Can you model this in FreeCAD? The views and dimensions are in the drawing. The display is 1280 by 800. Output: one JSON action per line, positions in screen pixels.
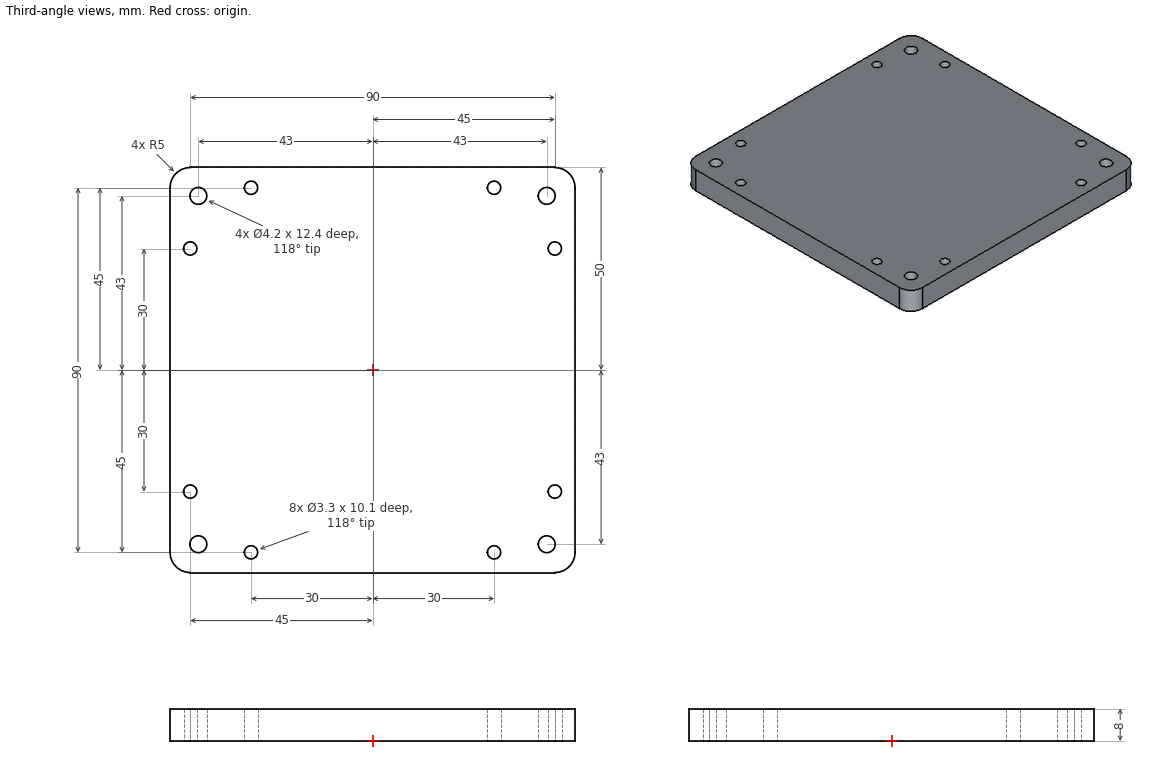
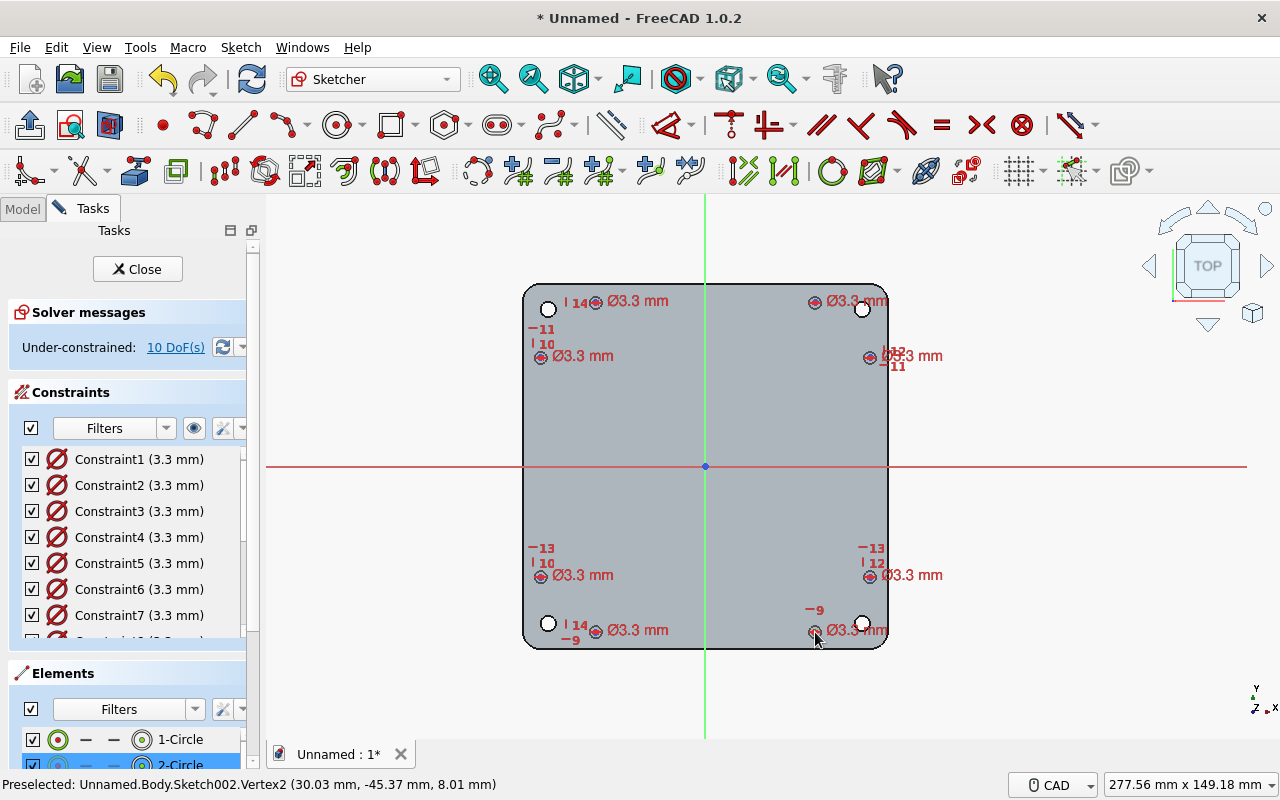
{"action": "left_click", "coordinate": [815, 303]}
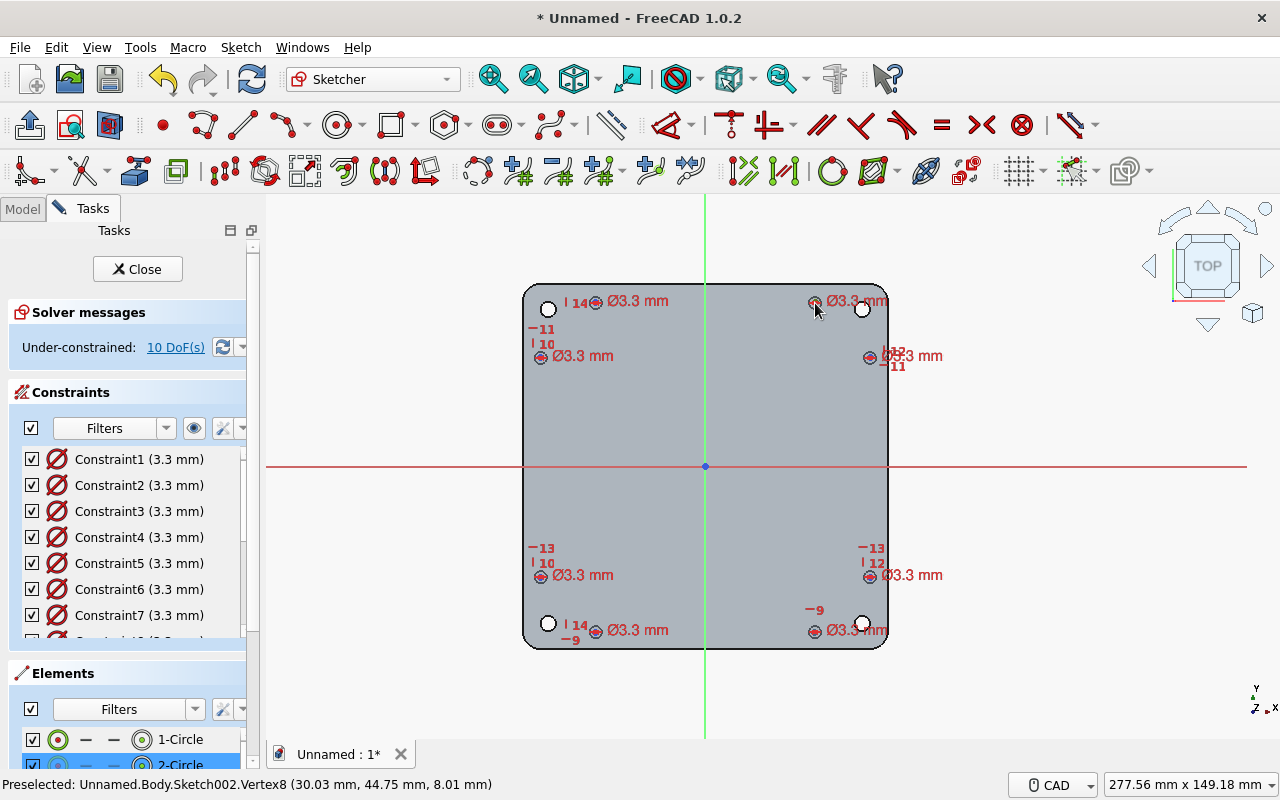
{"action": "key", "text": "v"}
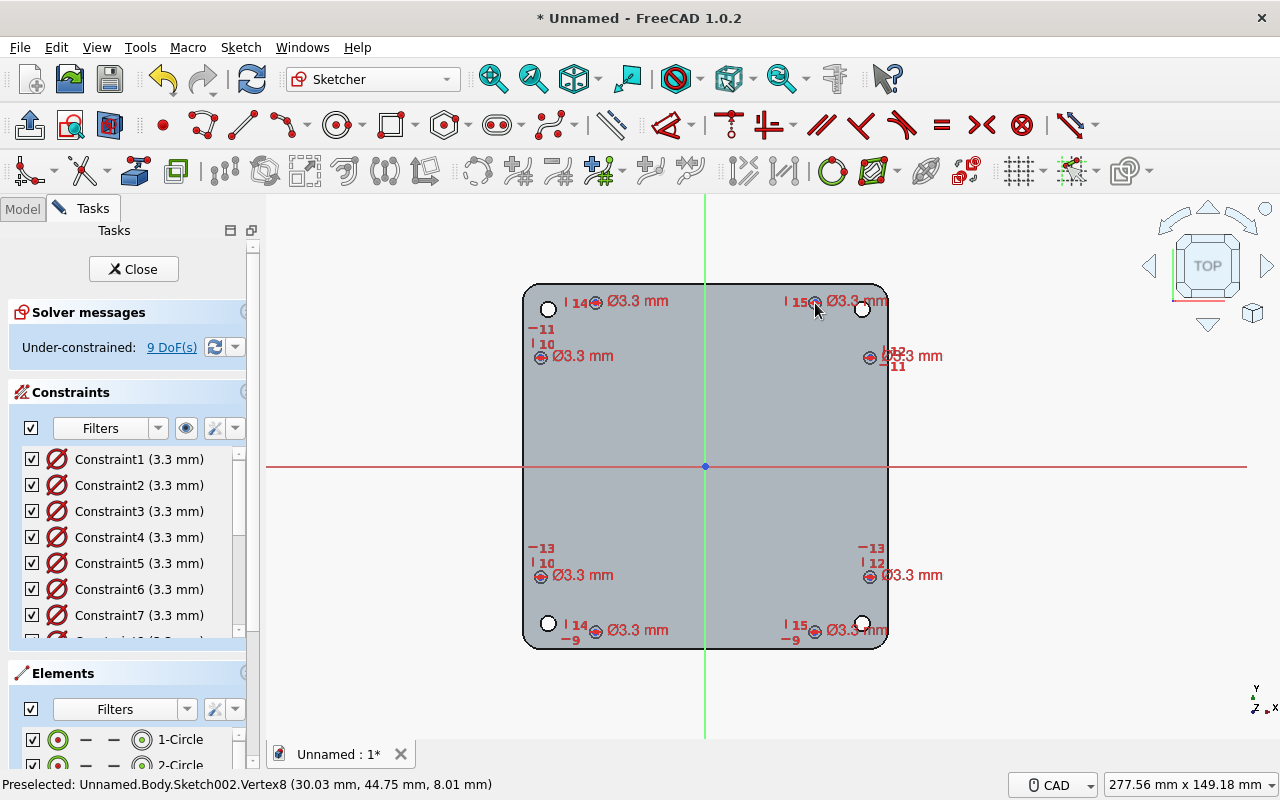
{"action": "left_click", "coordinate": [596, 303]}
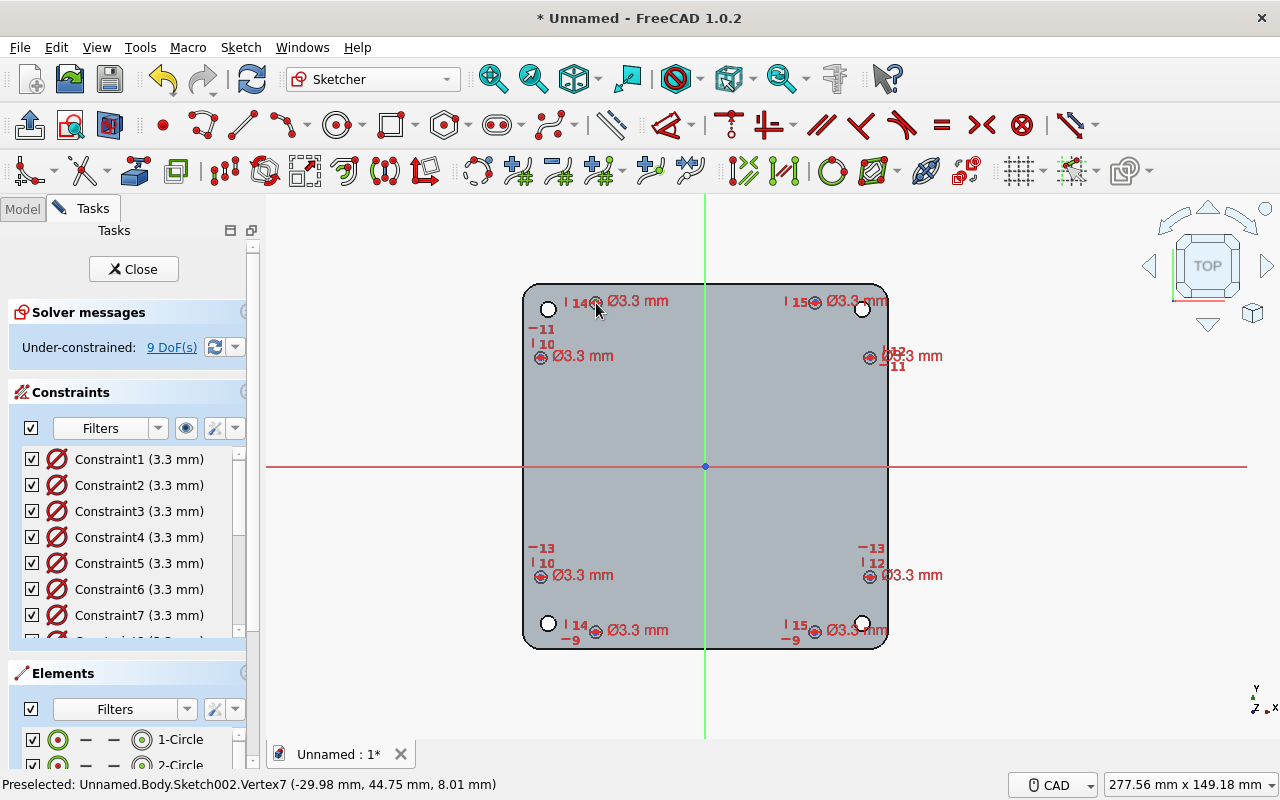
{"action": "left_click", "coordinate": [815, 303]}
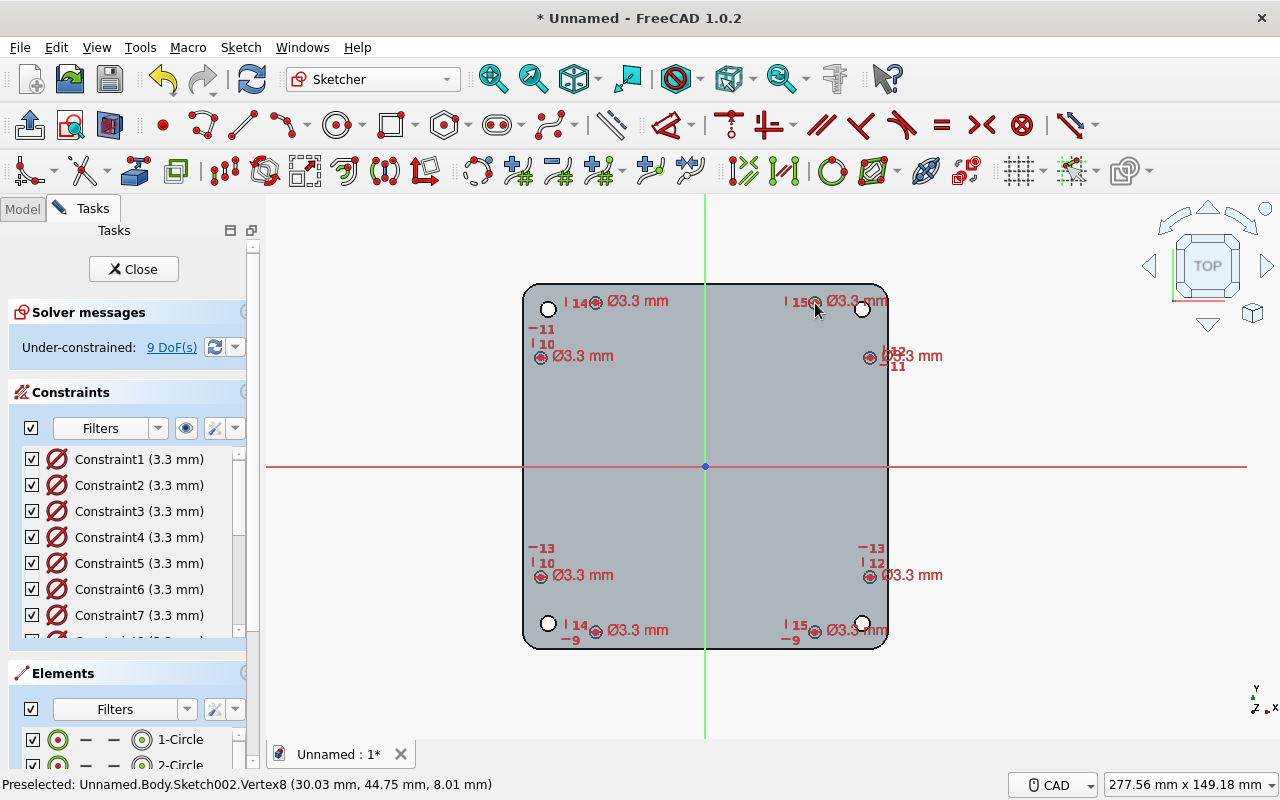
{"action": "key", "text": "h"}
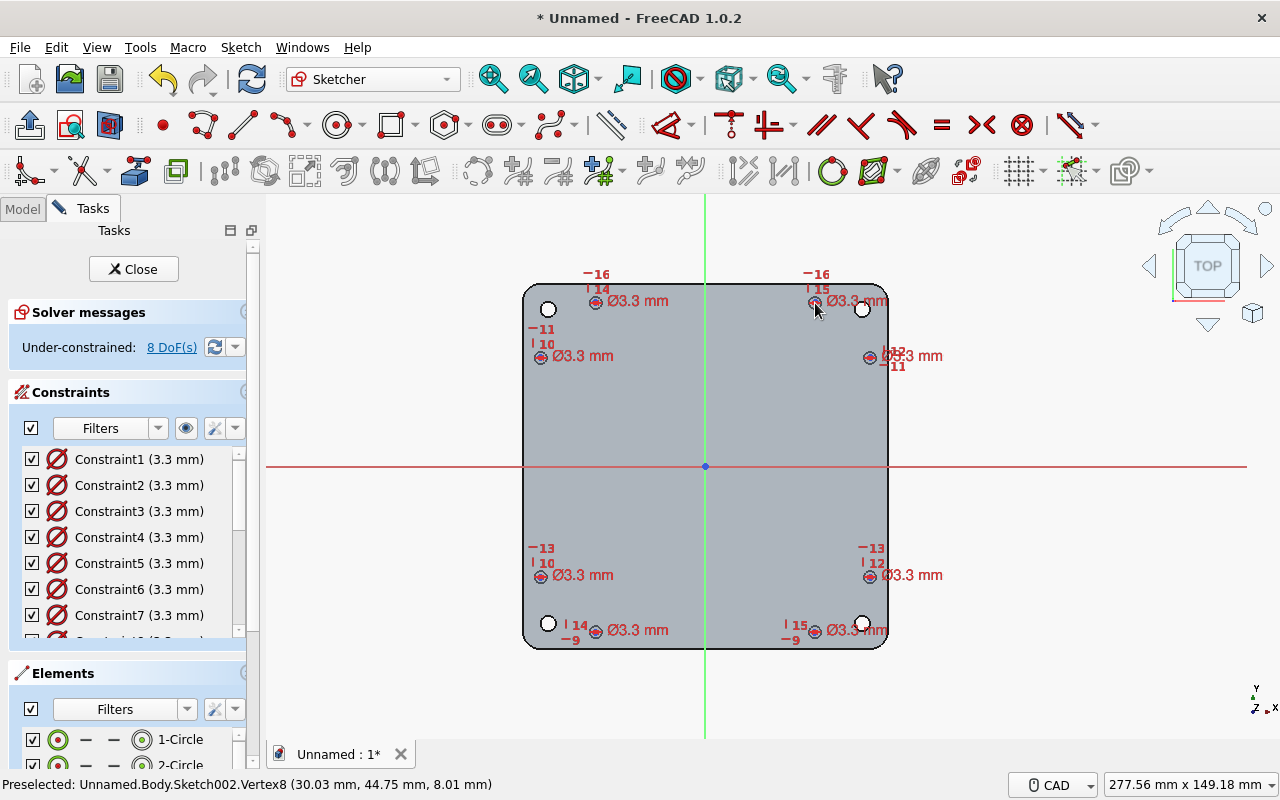
{"action": "key", "text": "d"}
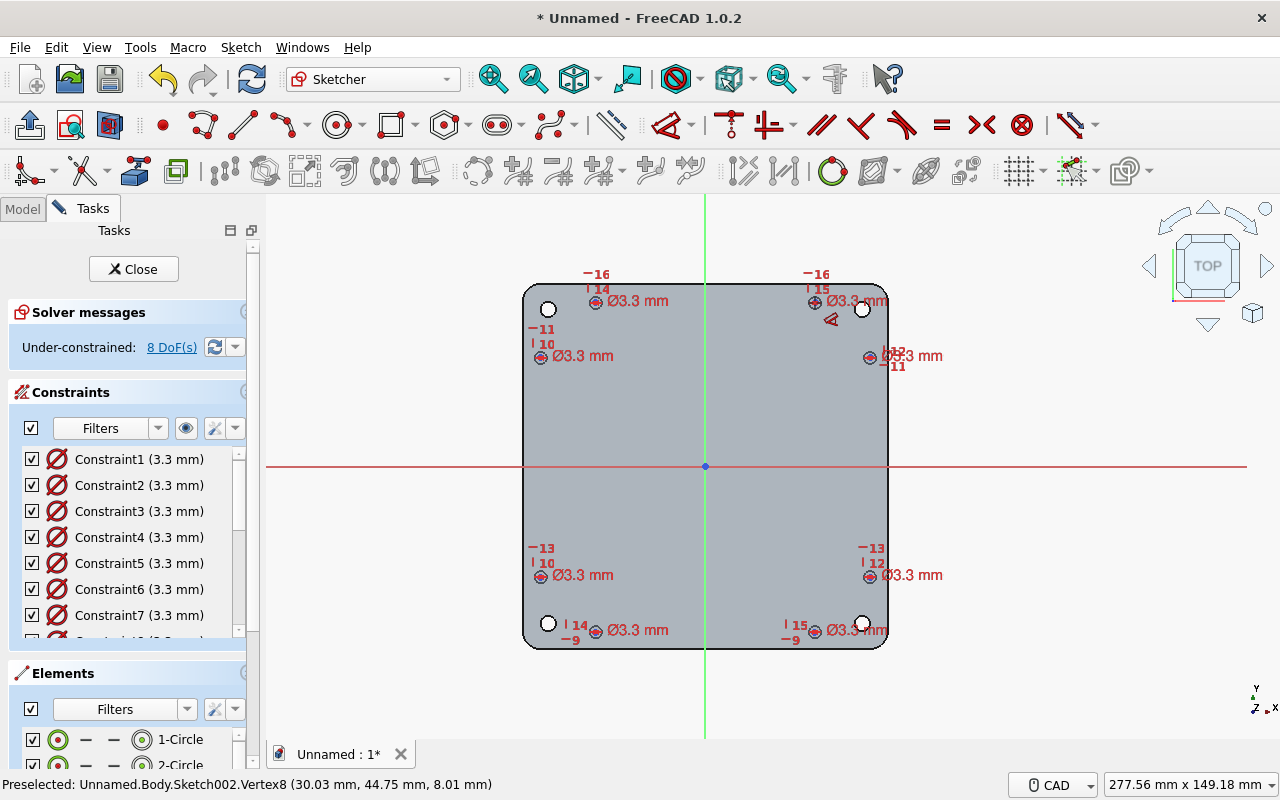
{"action": "left_click", "coordinate": [596, 632]}
{"action": "left_click", "coordinate": [651, 666]}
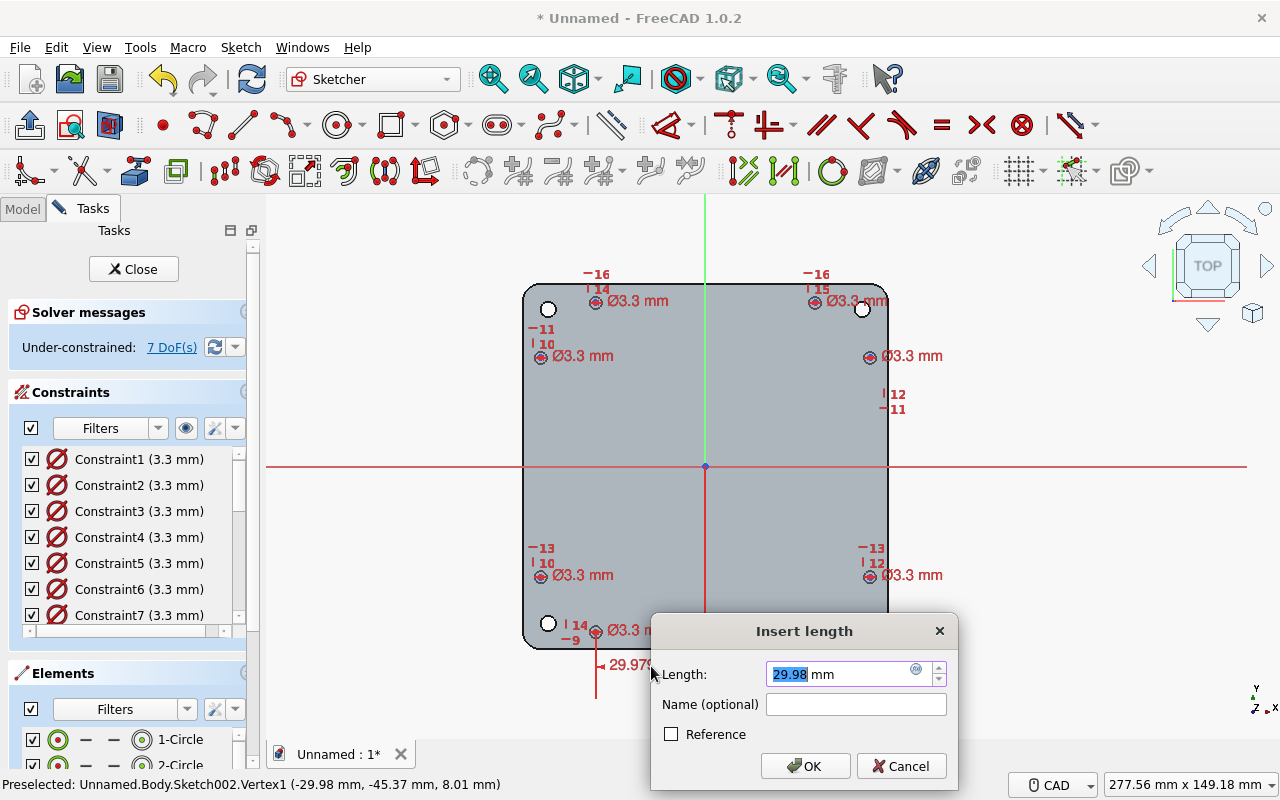
{"action": "type", "text": "30"}
{"action": "key", "text": "Return"}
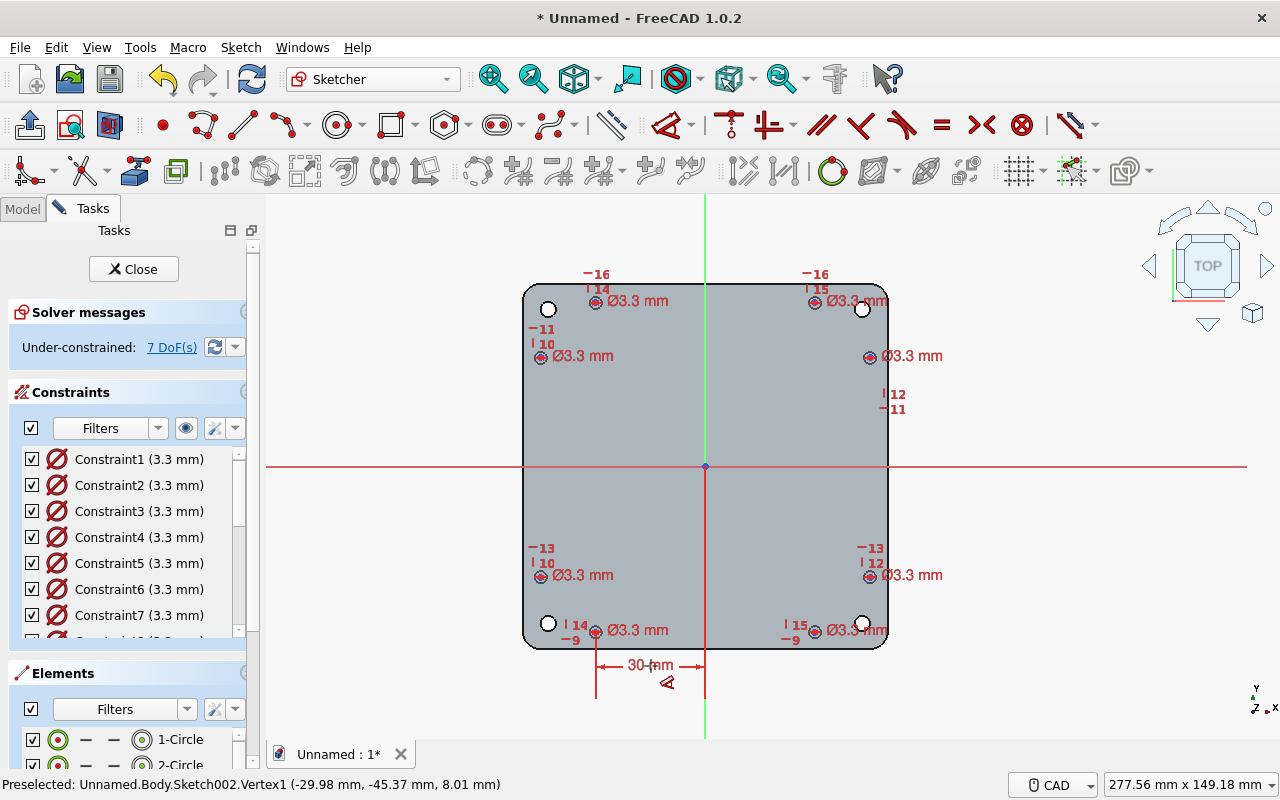
{"action": "left_click", "coordinate": [596, 632]}
{"action": "left_click", "coordinate": [562, 549]}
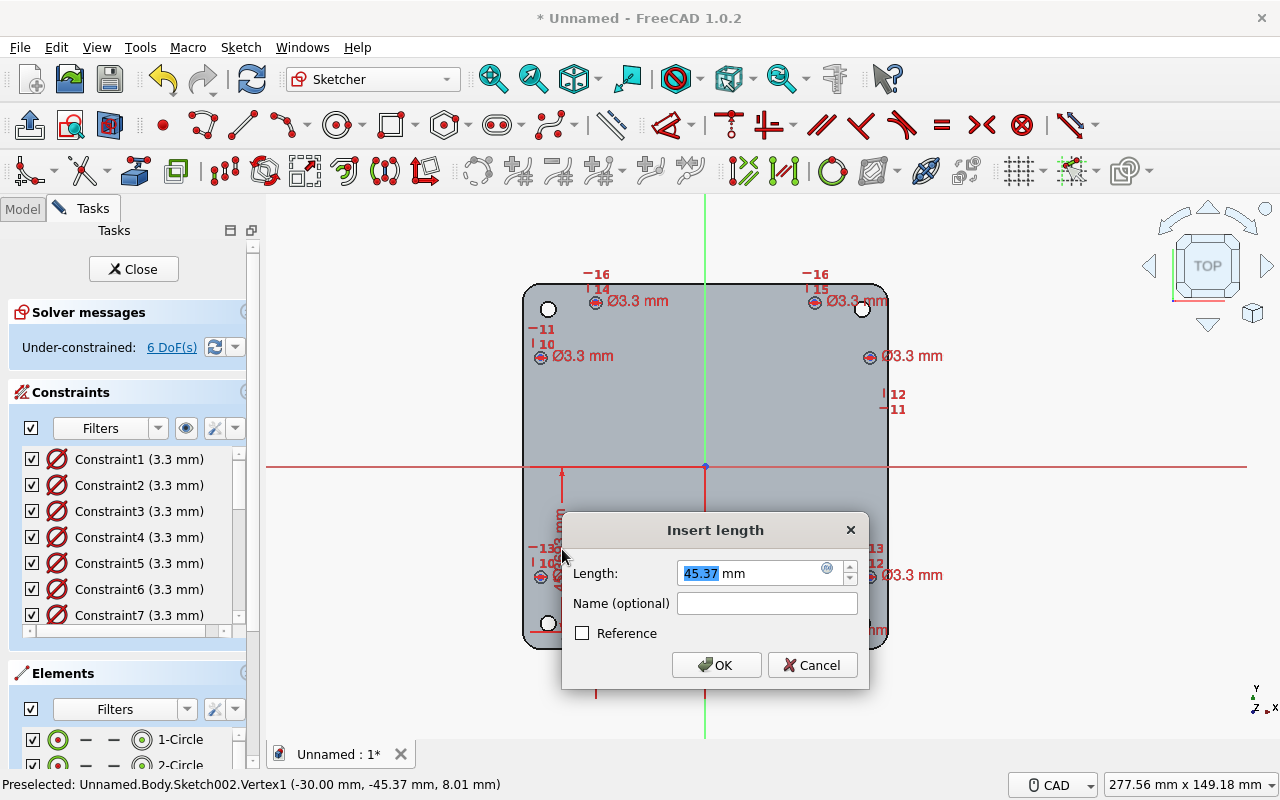
{"action": "type", "text": "45"}
{"action": "key", "text": "Return"}